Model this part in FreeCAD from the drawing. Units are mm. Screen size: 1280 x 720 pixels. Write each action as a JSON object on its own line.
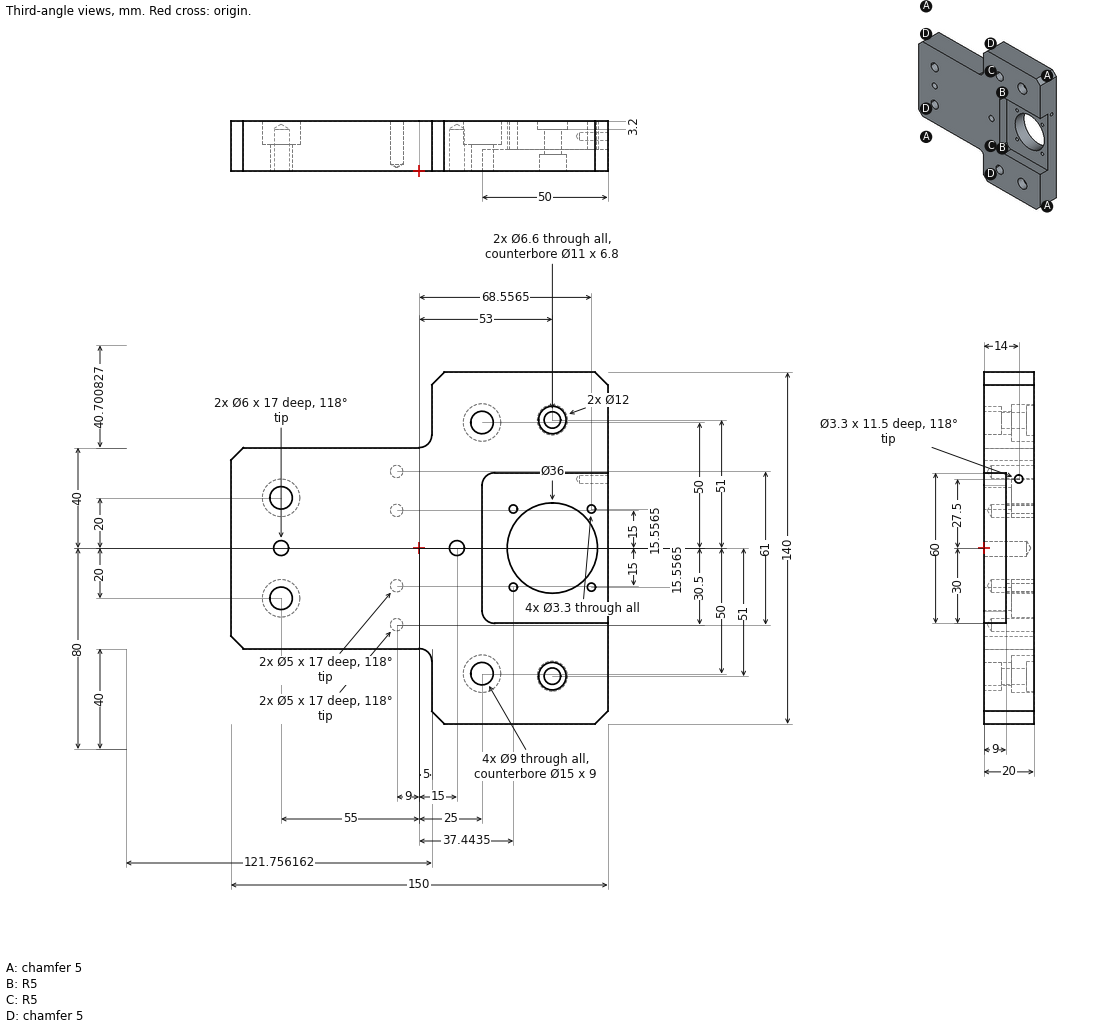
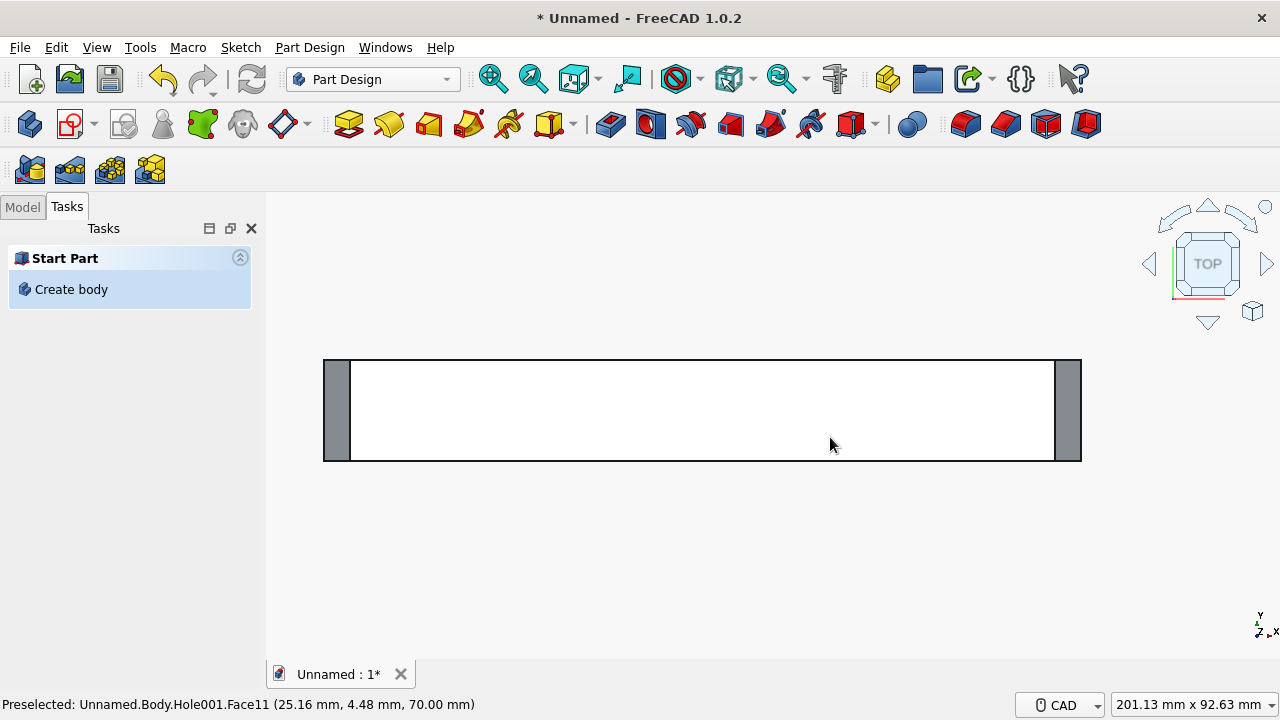
{"action": "left_click", "coordinate": [494, 80]}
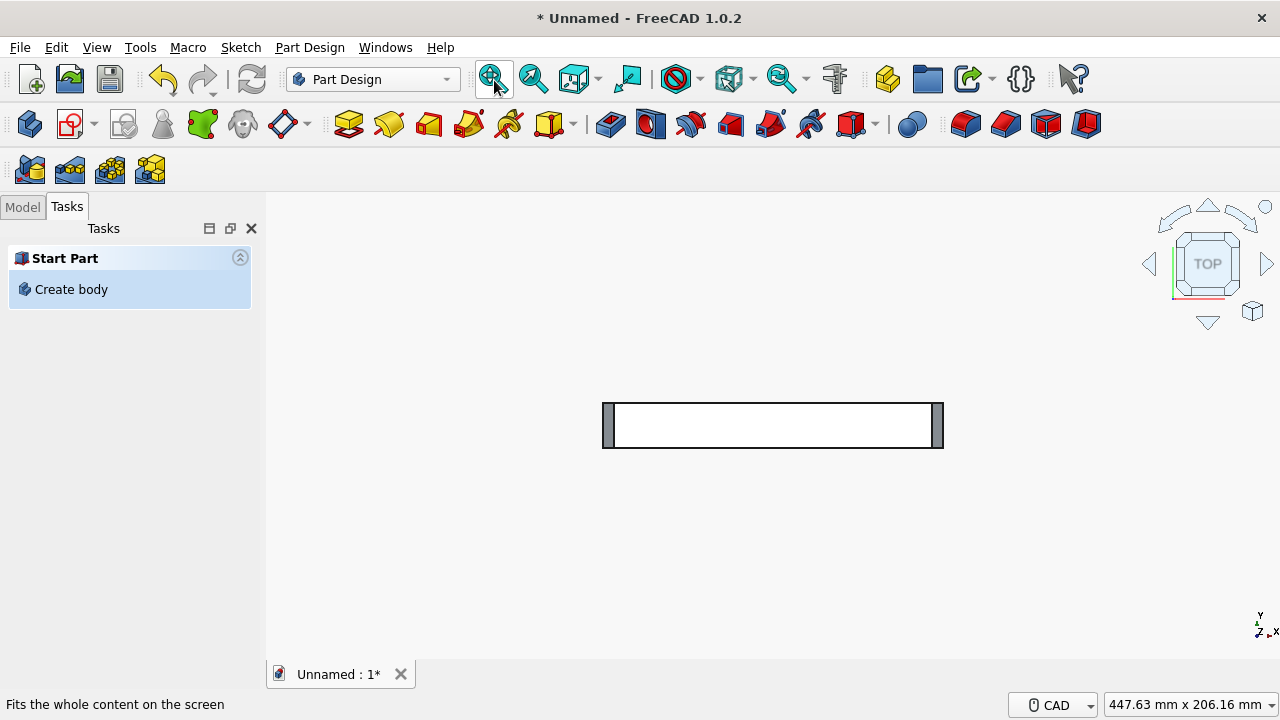
{"action": "key", "text": "0"}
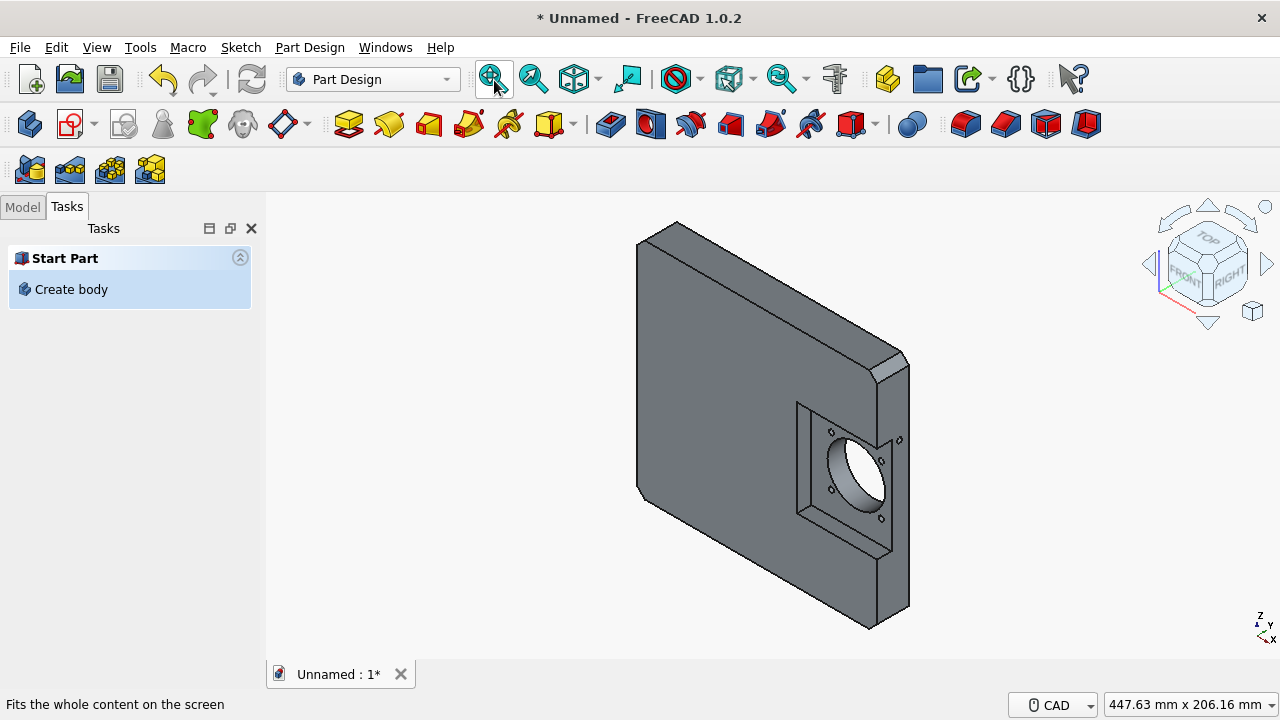
{"action": "scroll", "coordinate": [804, 397], "scroll_direction": "up", "scroll_amount": 4}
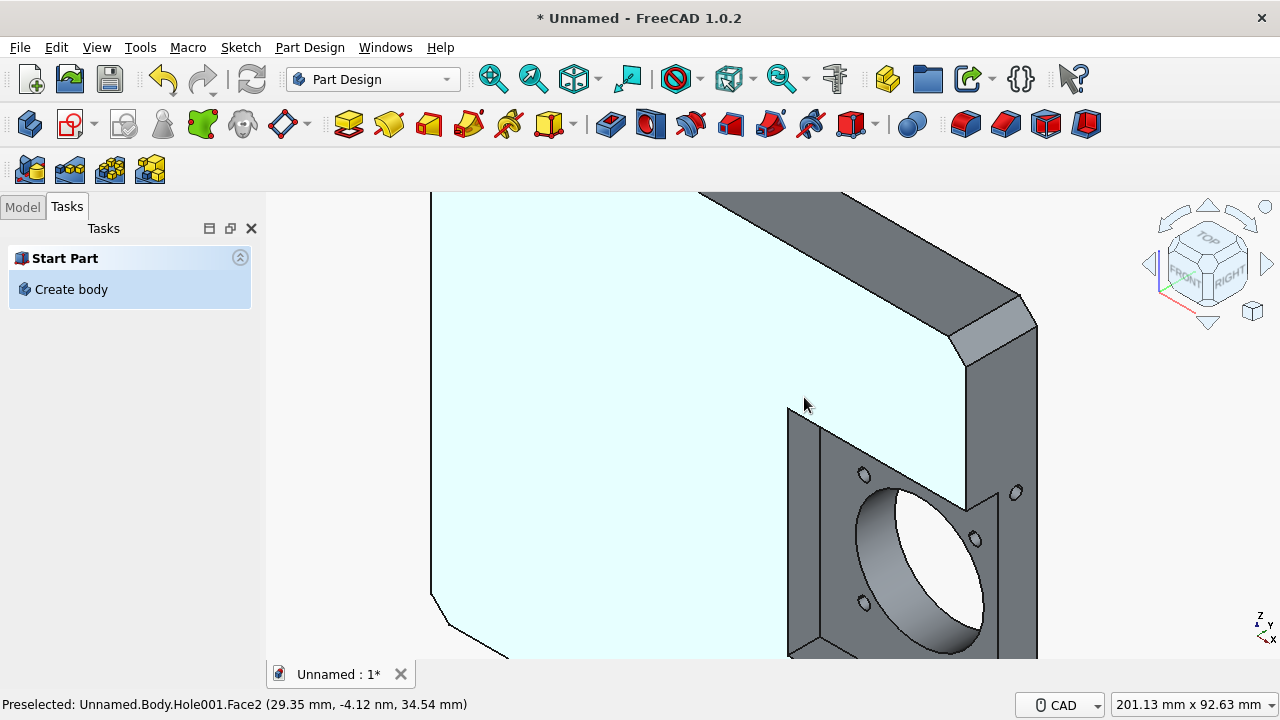
{"action": "left_click", "coordinate": [494, 80]}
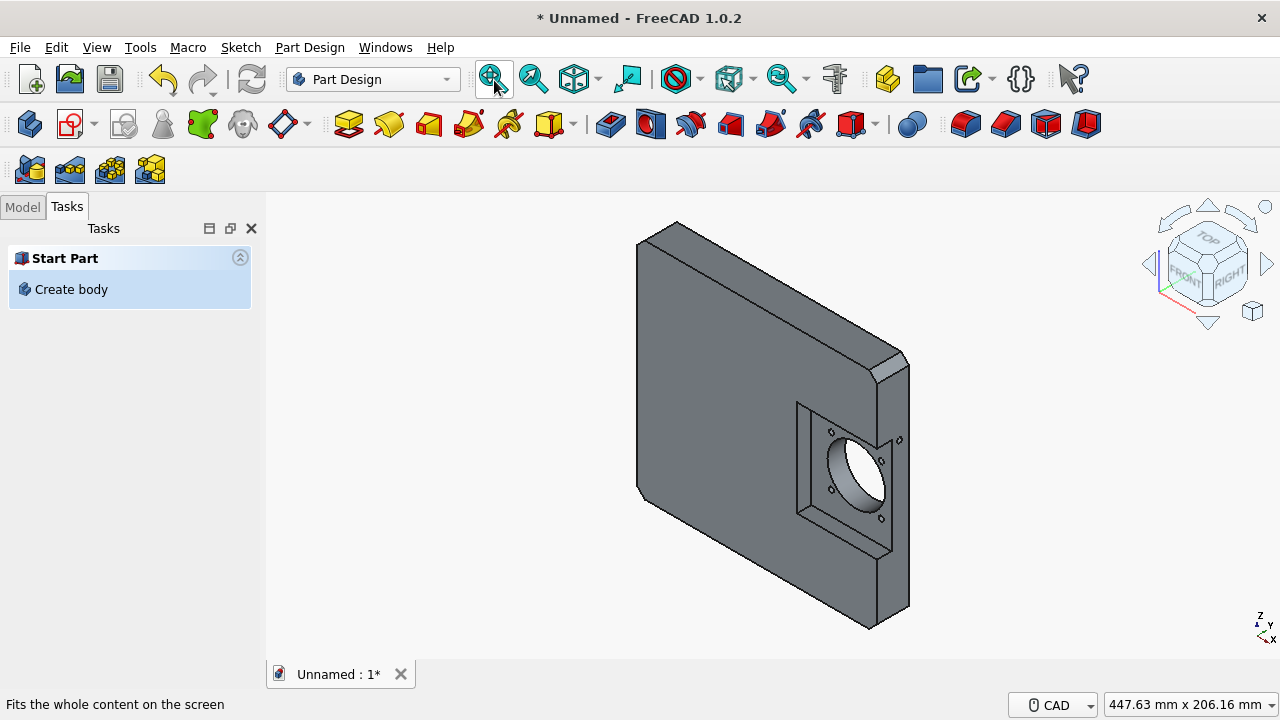
{"action": "key", "text": "1"}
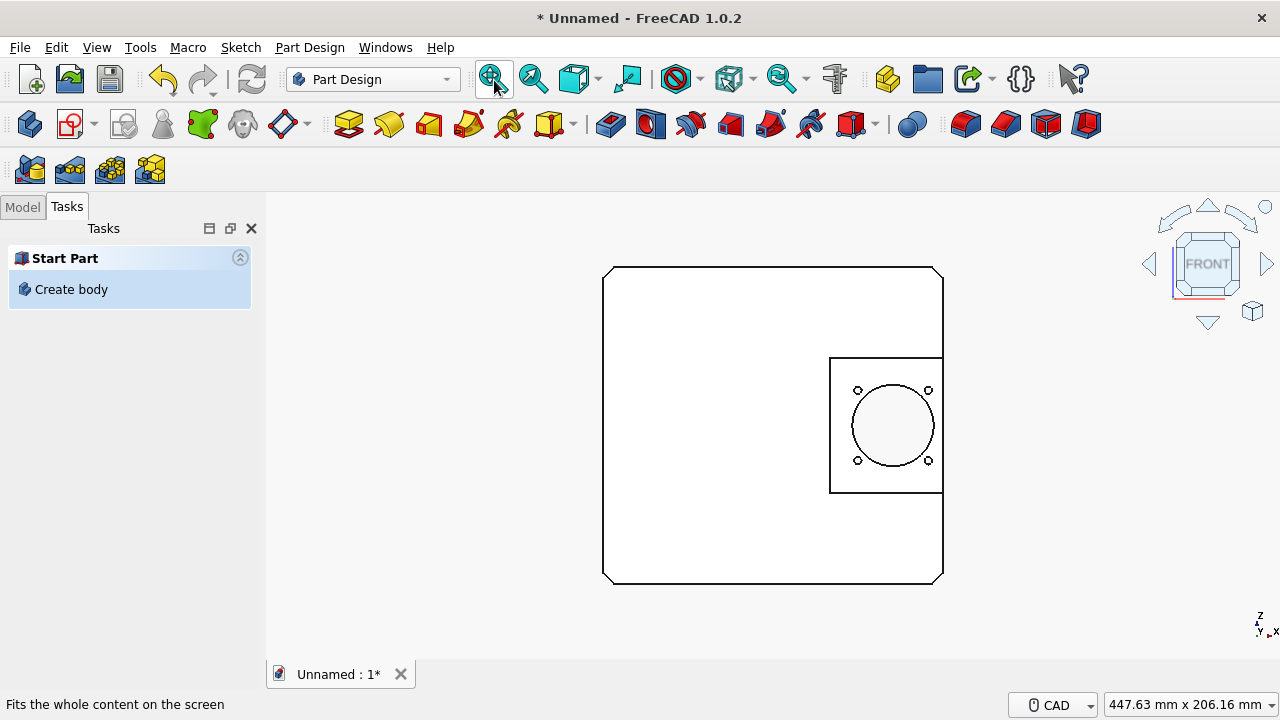
{"action": "scroll", "coordinate": [830, 357], "scroll_direction": "up", "scroll_amount": 4}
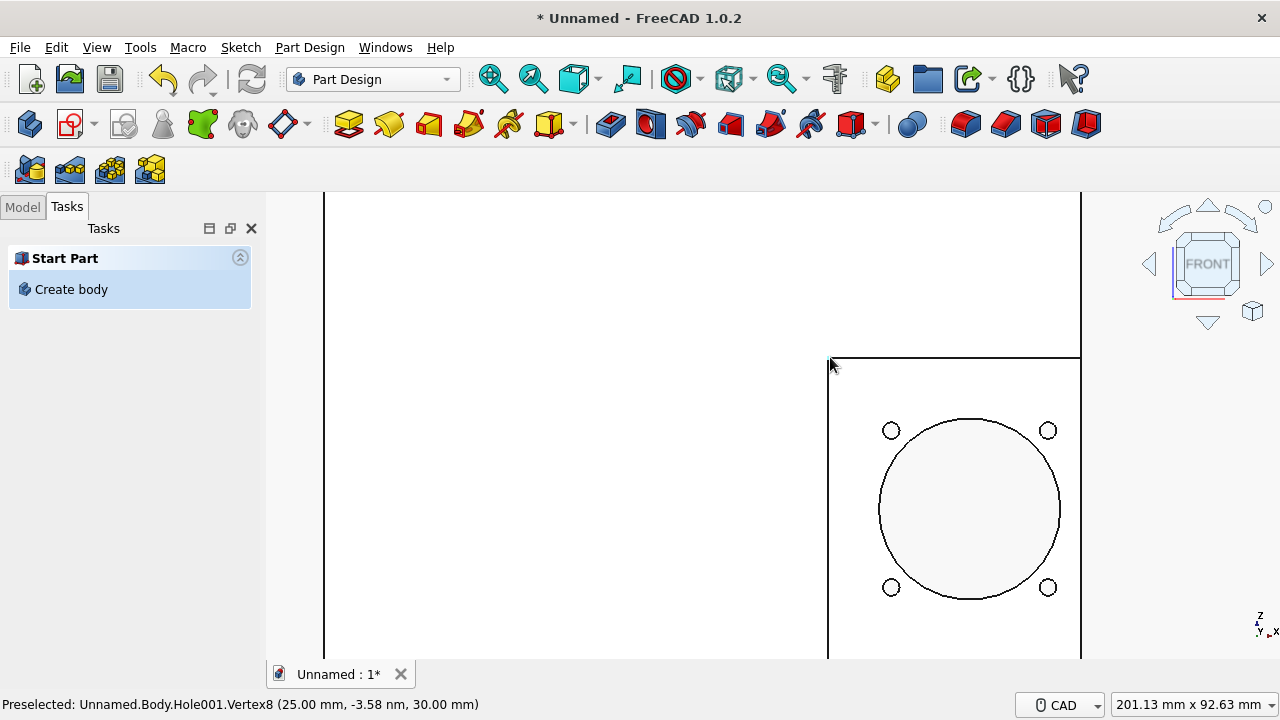
{"action": "left_click", "coordinate": [494, 80]}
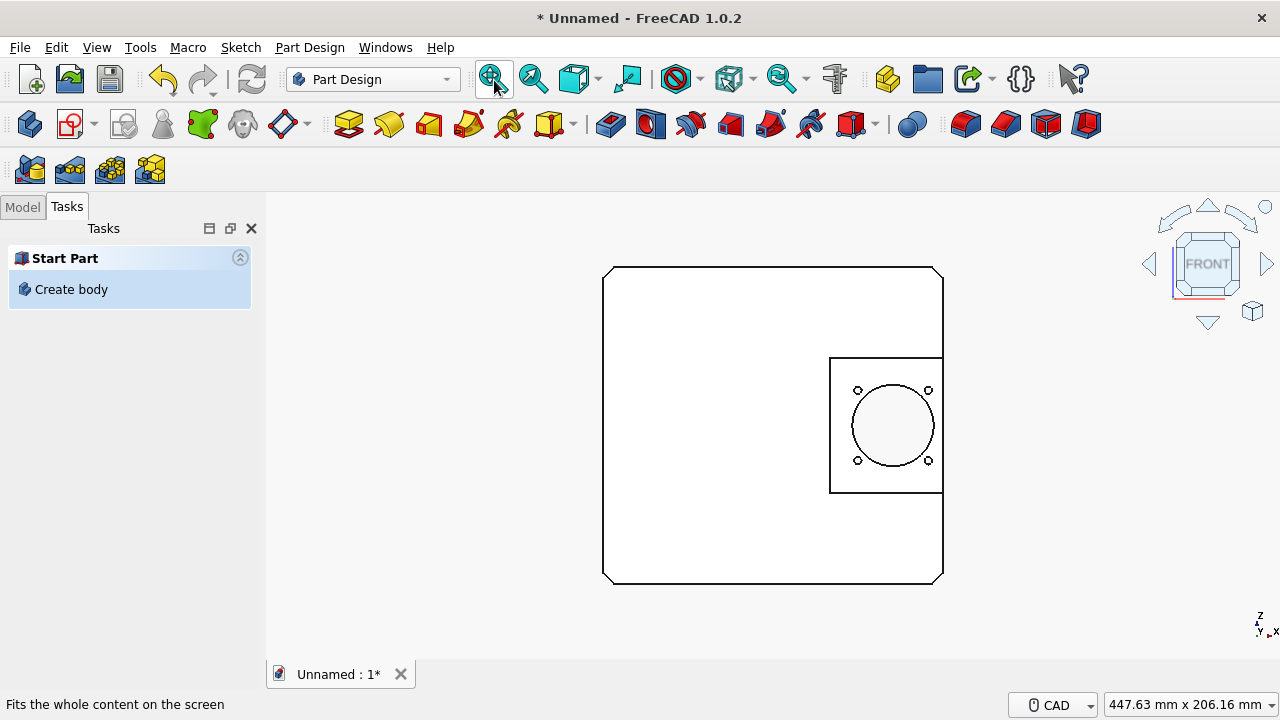
{"action": "key", "text": "3"}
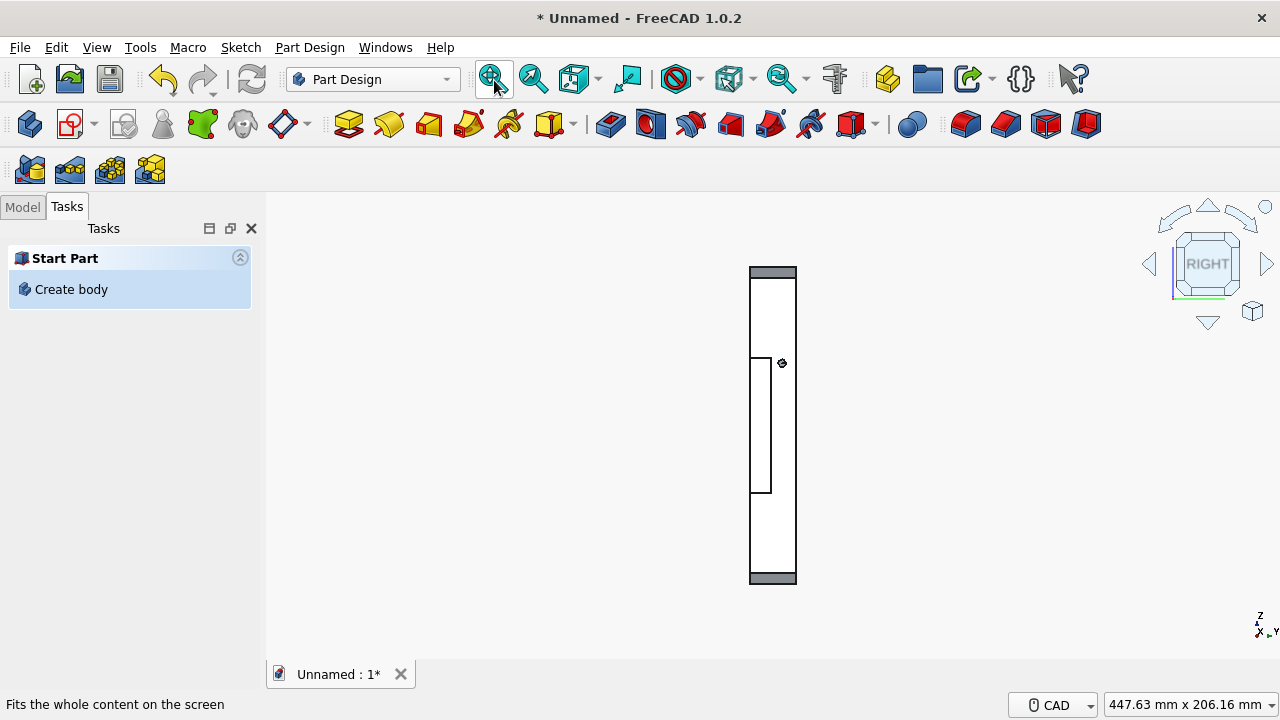
{"action": "scroll", "coordinate": [761, 357], "scroll_direction": "up", "scroll_amount": 4}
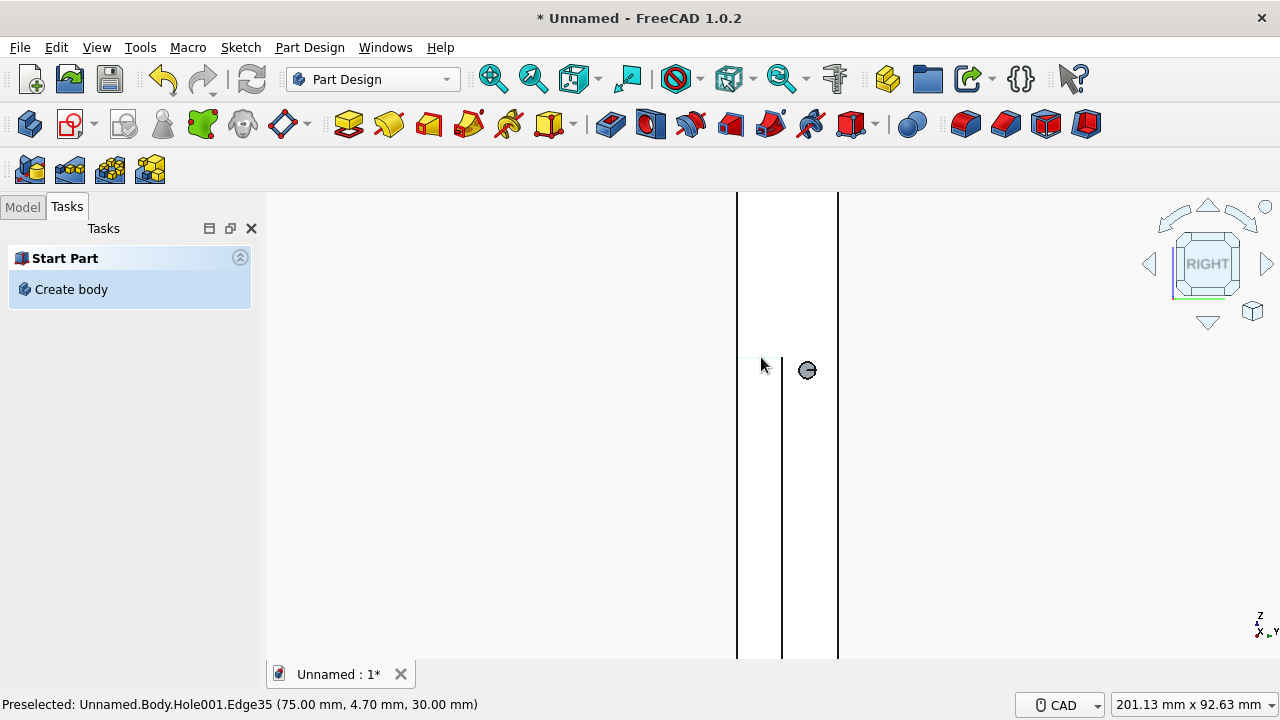
{"action": "left_click", "coordinate": [494, 80]}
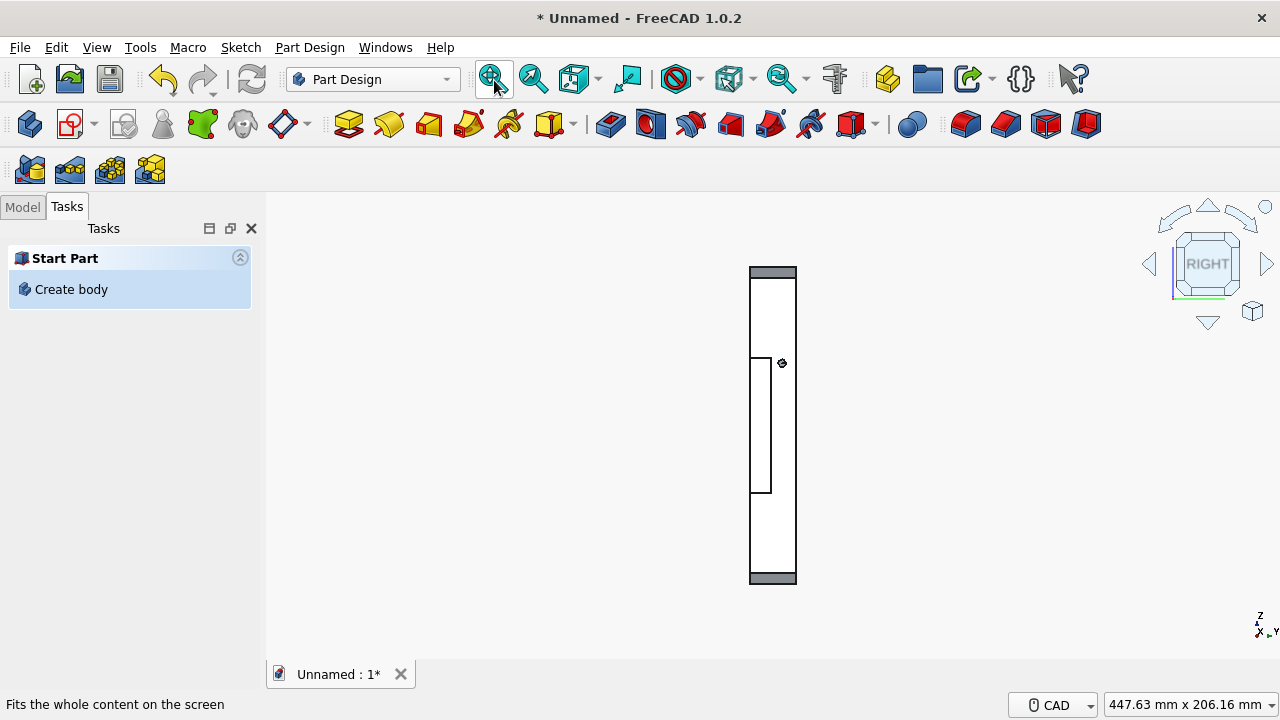
{"action": "key", "text": "5"}